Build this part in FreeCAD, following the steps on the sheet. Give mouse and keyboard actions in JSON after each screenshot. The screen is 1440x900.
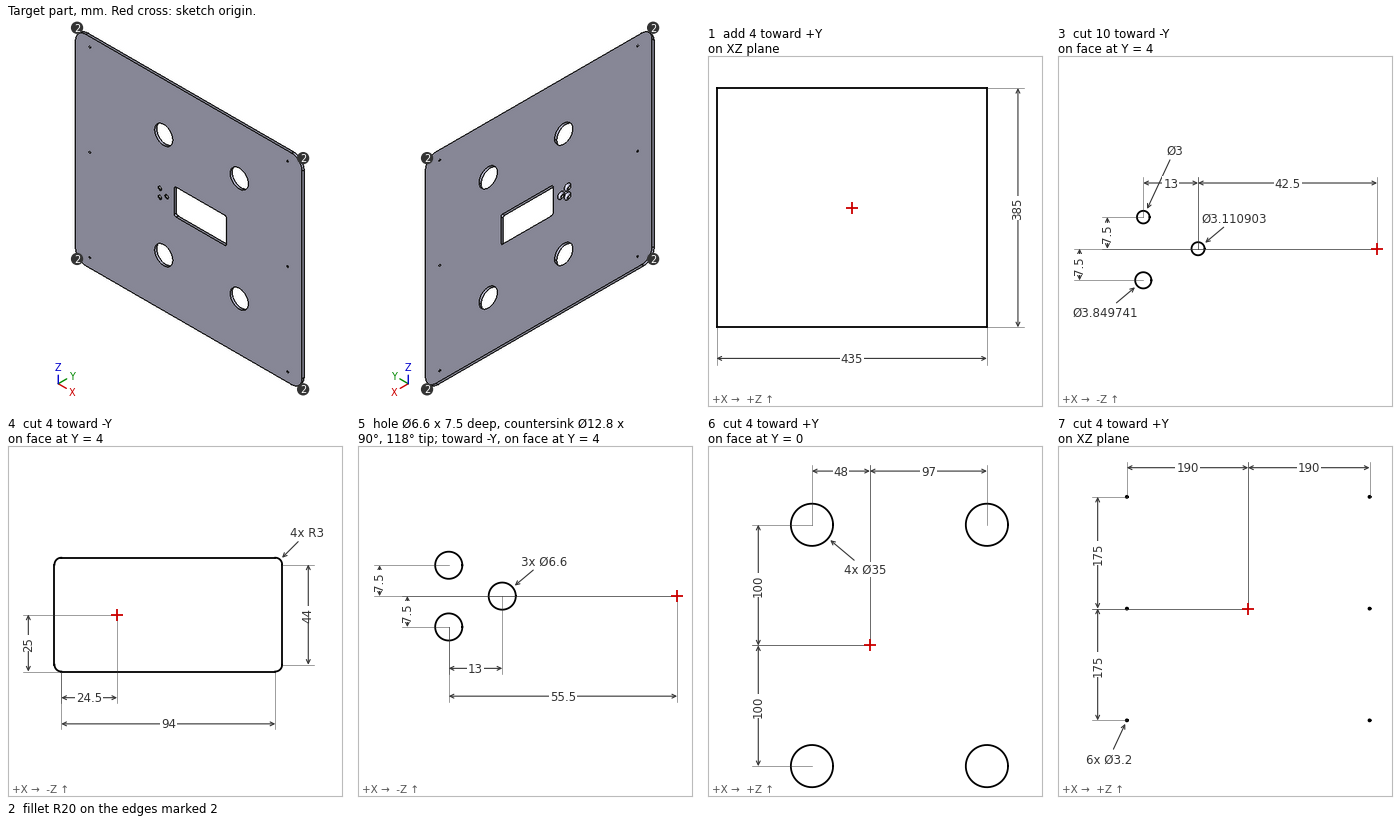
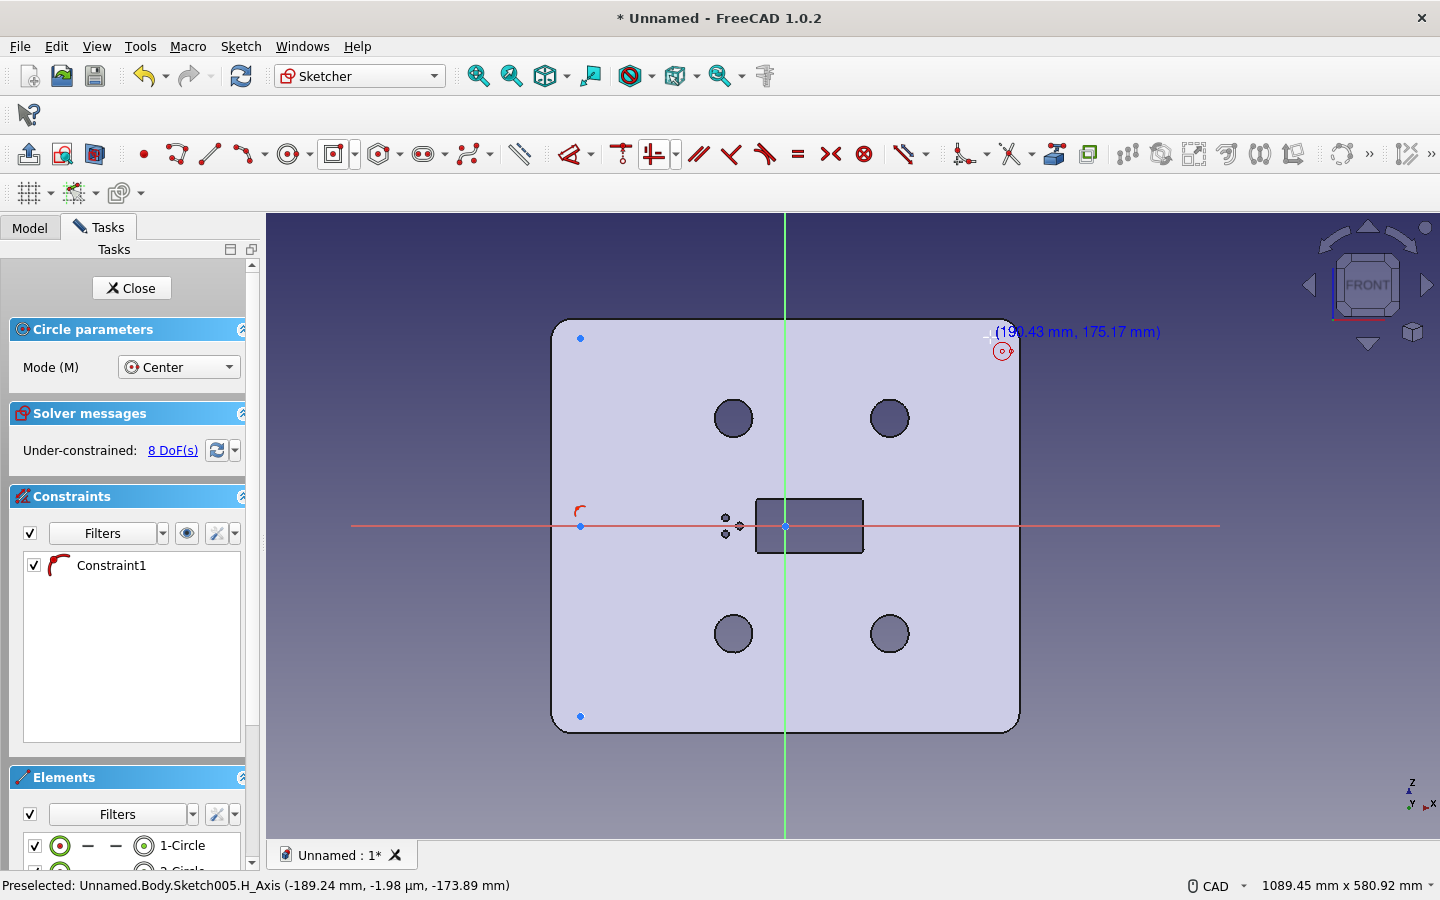
{"action": "left_click", "coordinate": [990, 337]}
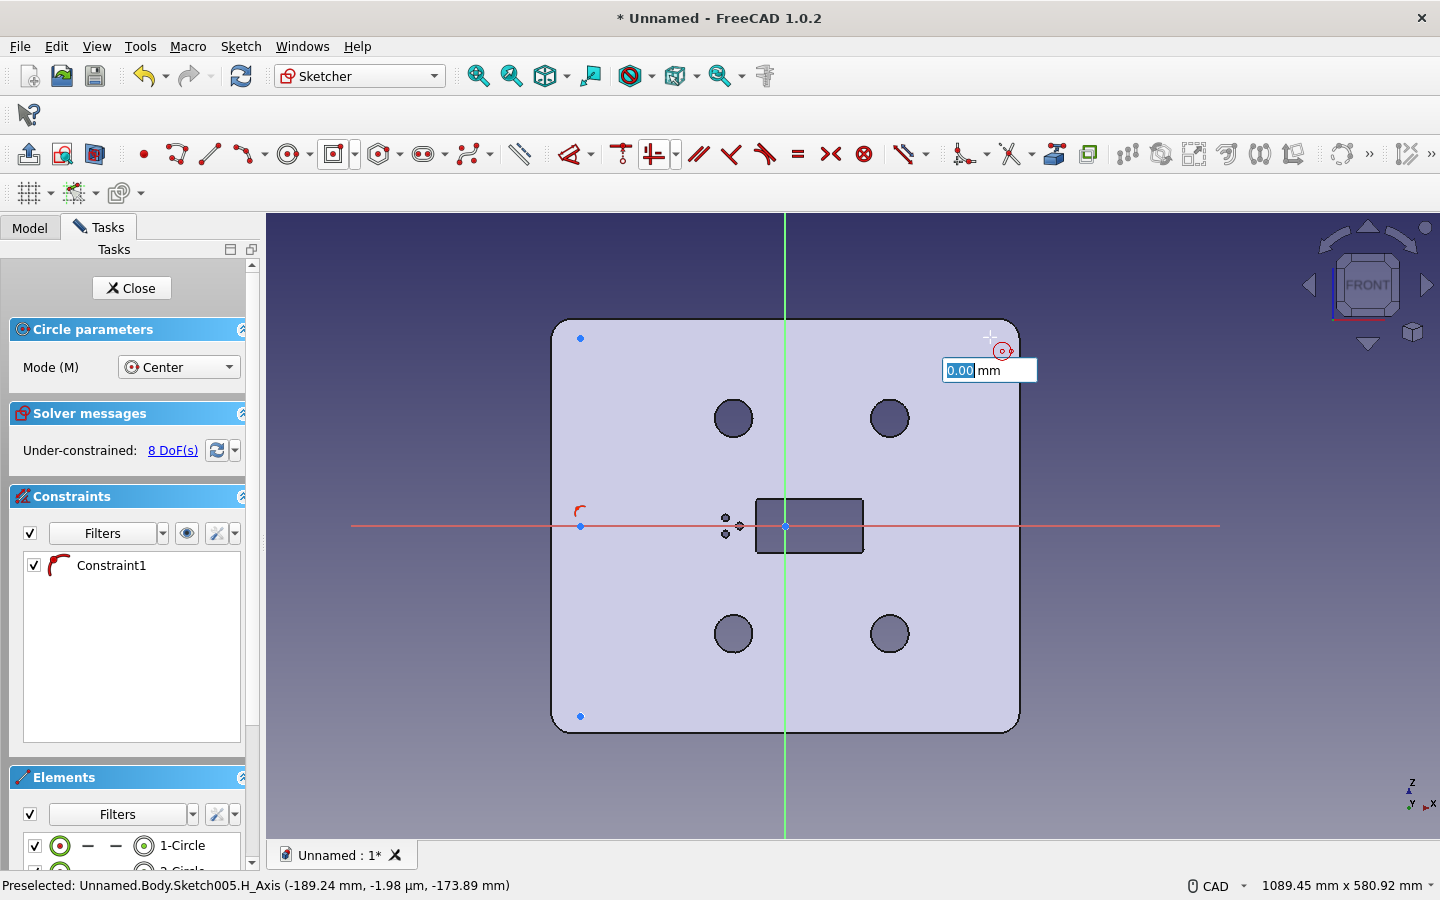
{"action": "scroll", "coordinate": [991, 336], "scroll_direction": "up", "scroll_amount": 12}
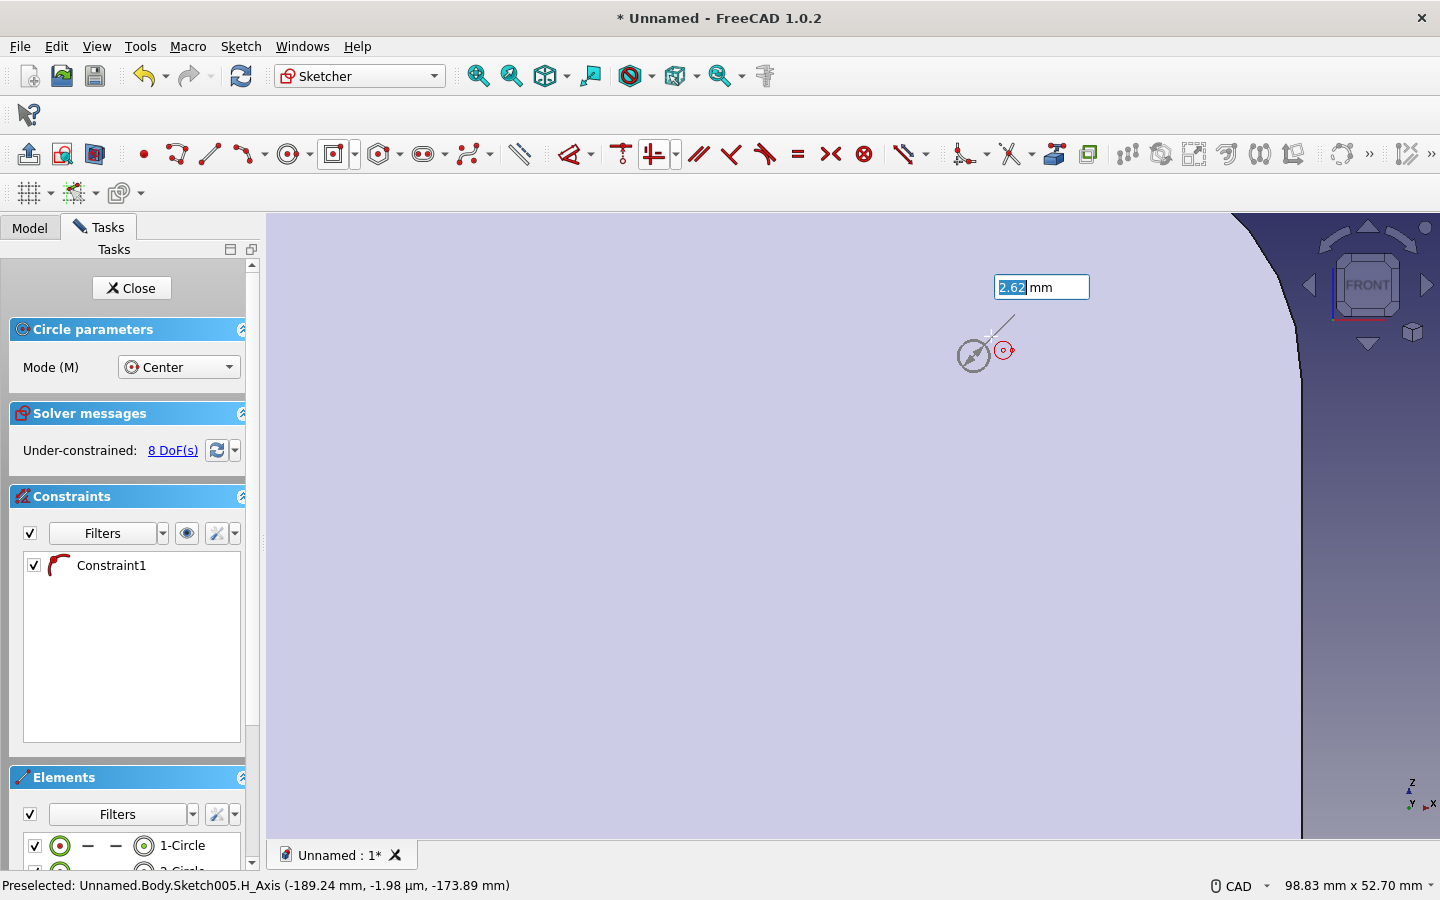
{"action": "left_click", "coordinate": [988, 336]}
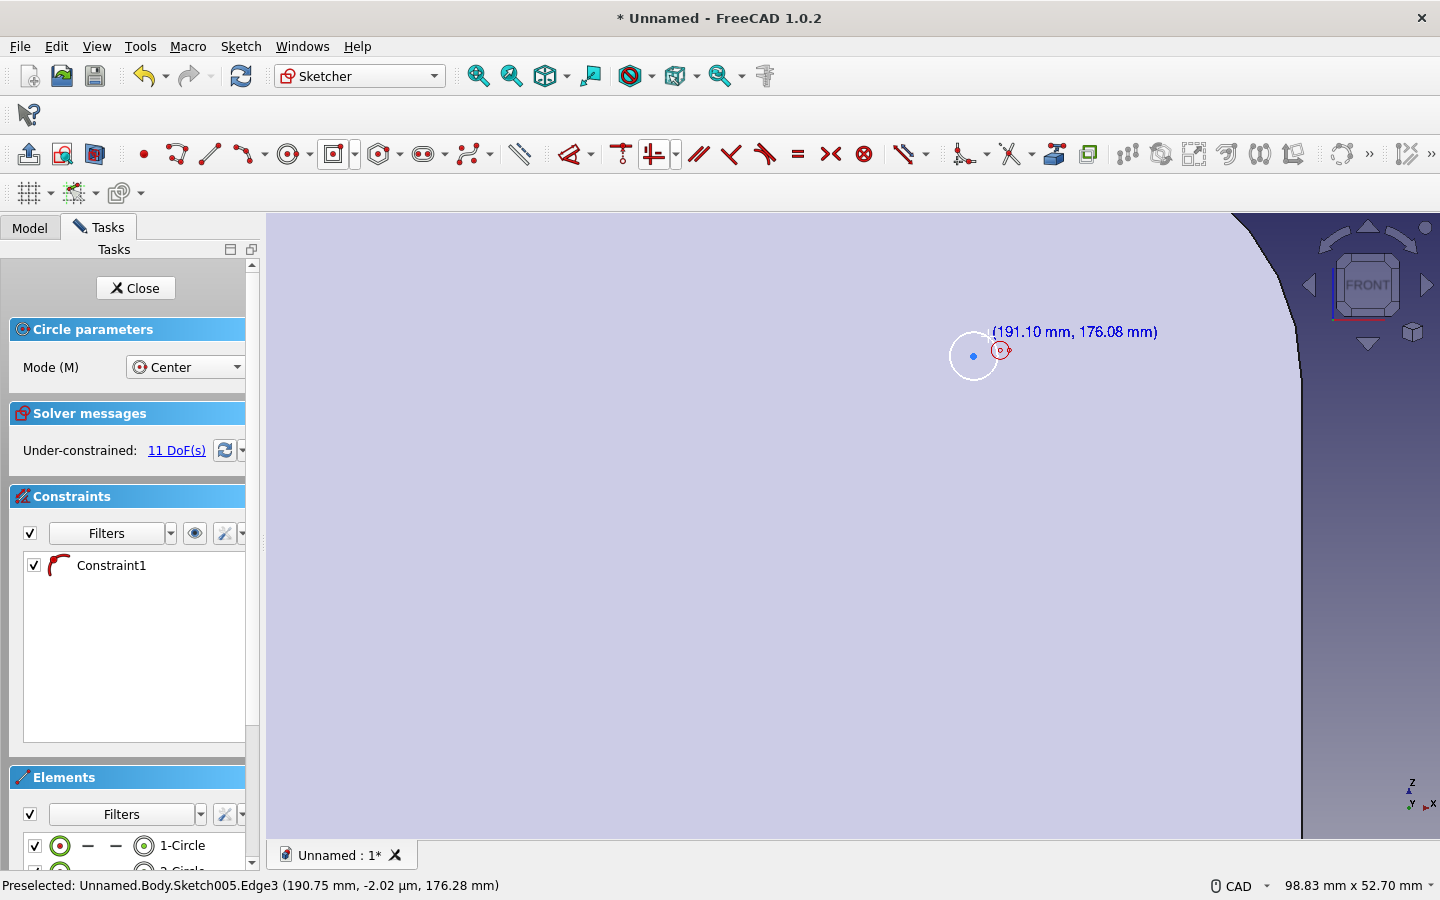
{"action": "scroll", "coordinate": [991, 336], "scroll_direction": "down", "scroll_amount": 12}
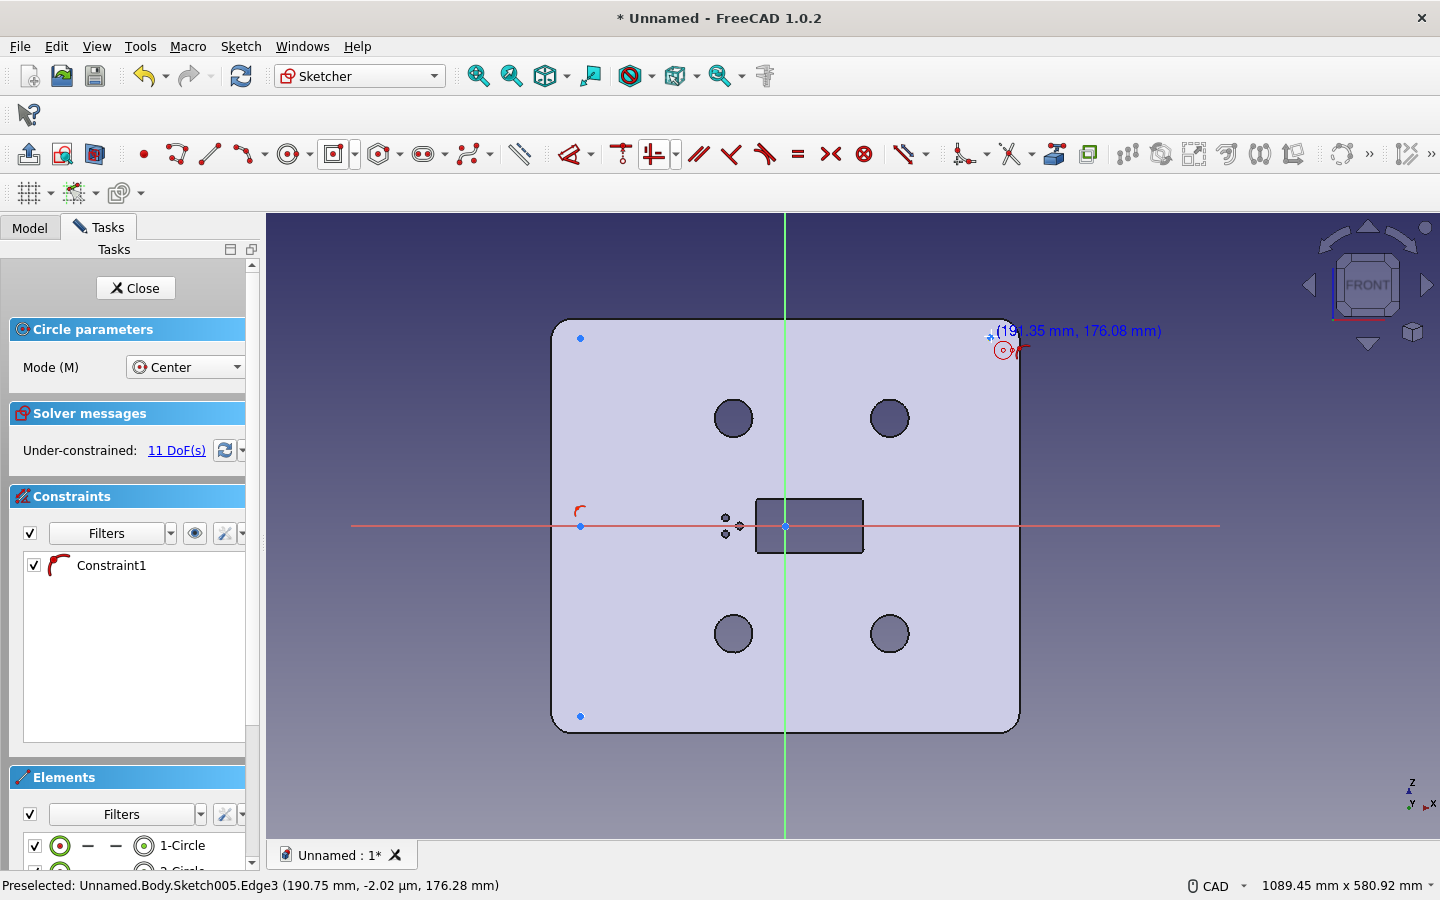
{"action": "scroll", "coordinate": [990, 526], "scroll_direction": "up", "scroll_amount": 13}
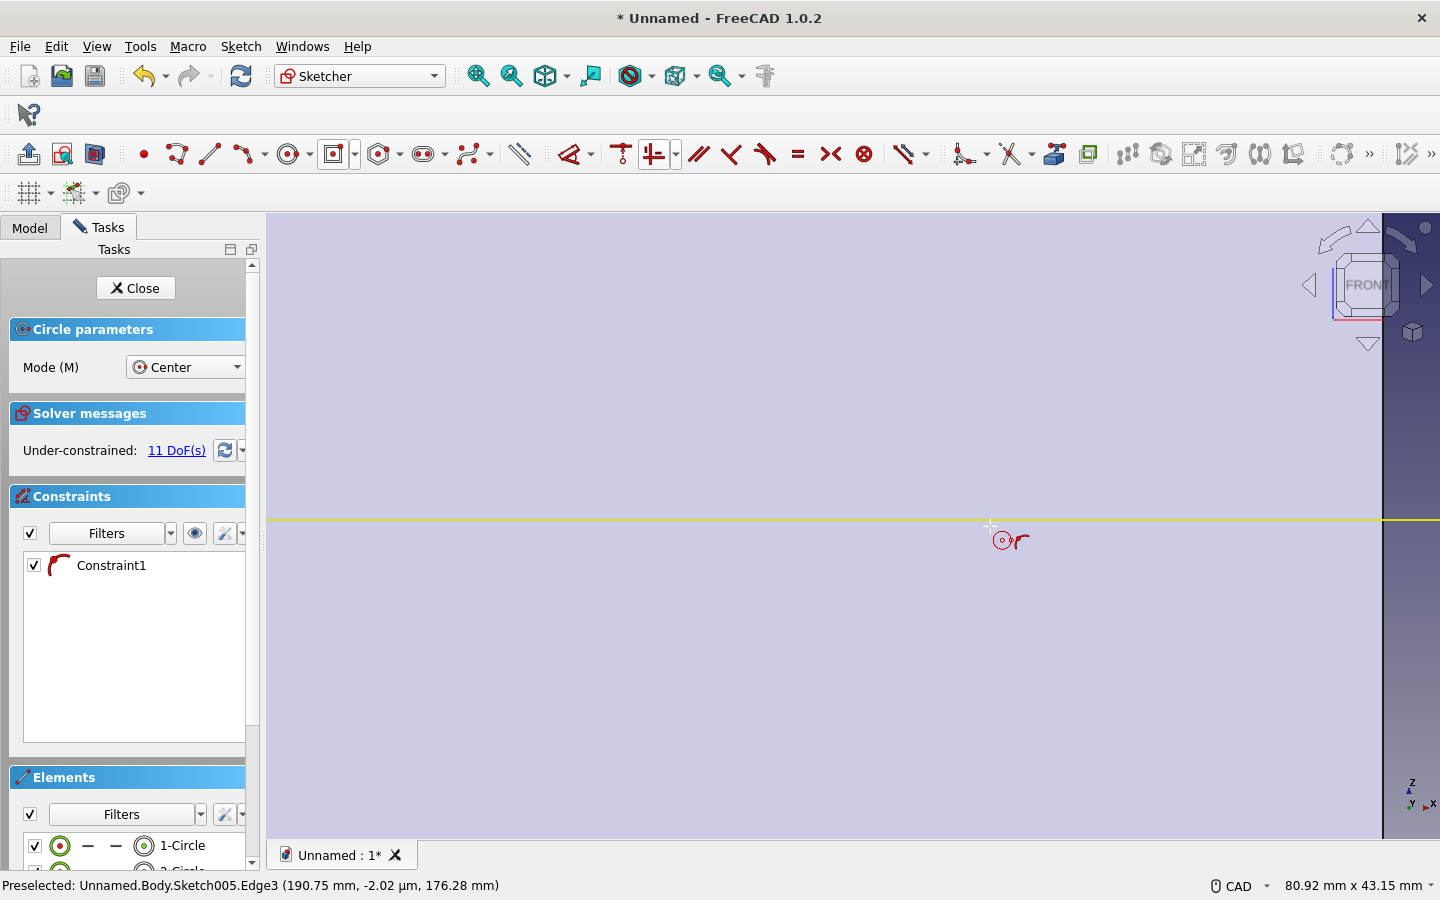
{"action": "scroll", "coordinate": [990, 526], "scroll_direction": "down", "scroll_amount": 13}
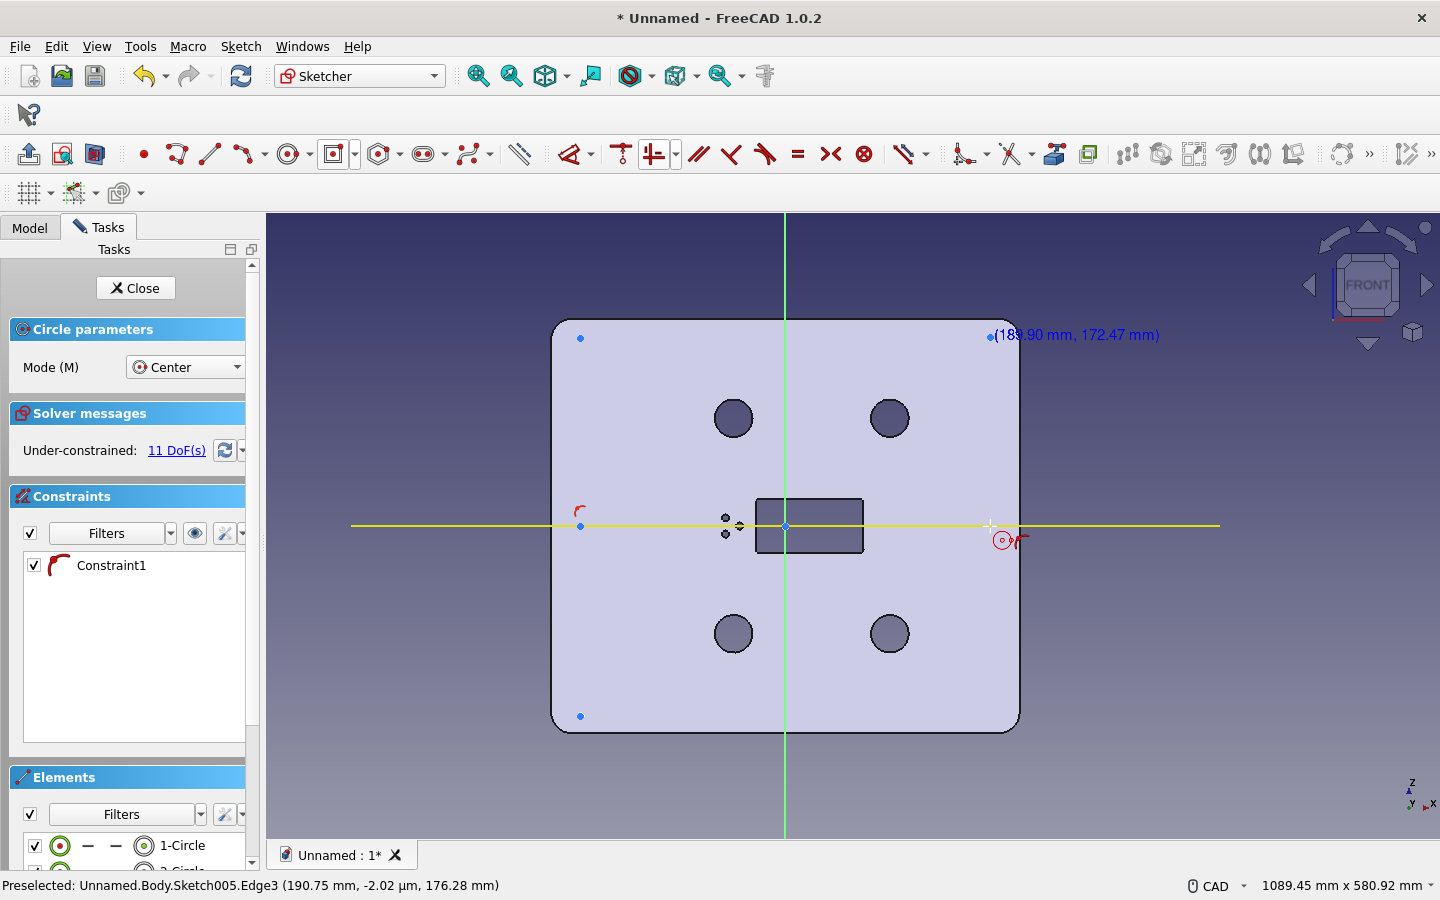
{"action": "left_click", "coordinate": [990, 526]}